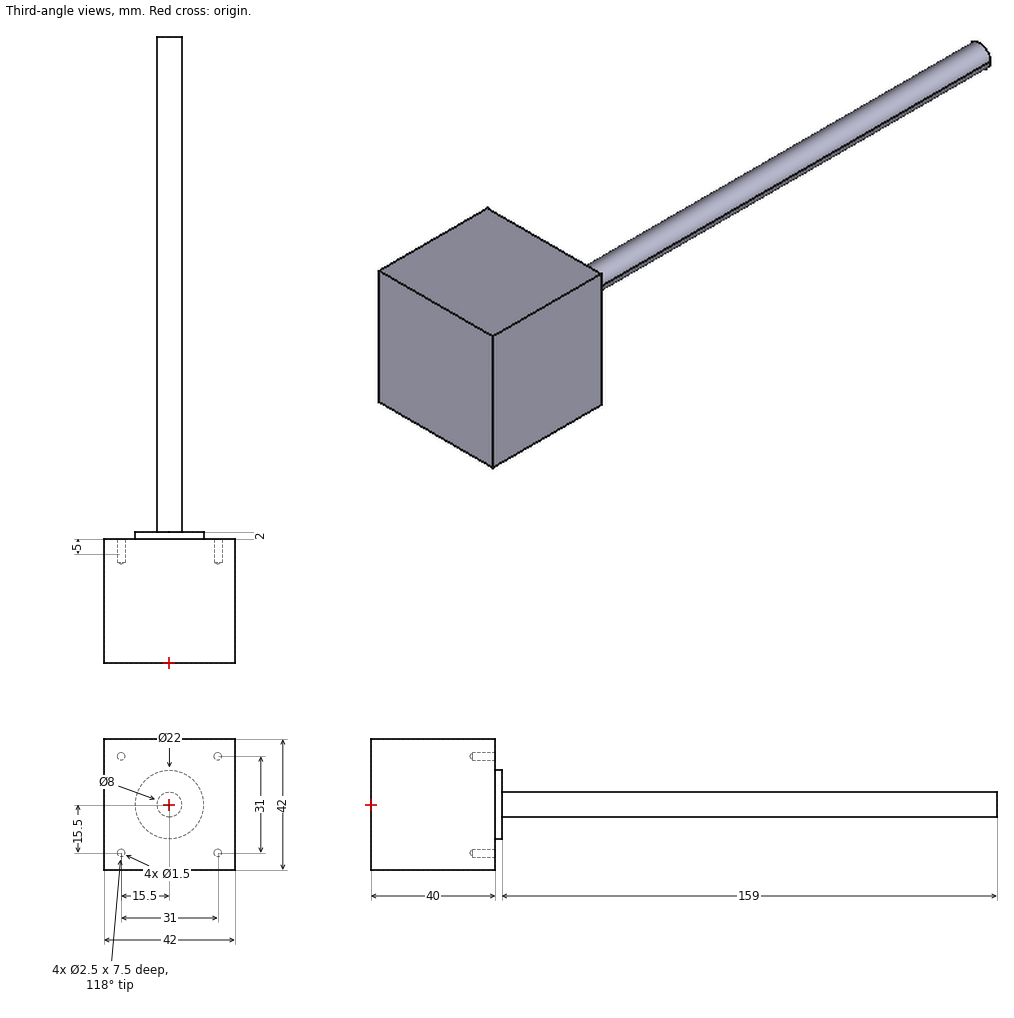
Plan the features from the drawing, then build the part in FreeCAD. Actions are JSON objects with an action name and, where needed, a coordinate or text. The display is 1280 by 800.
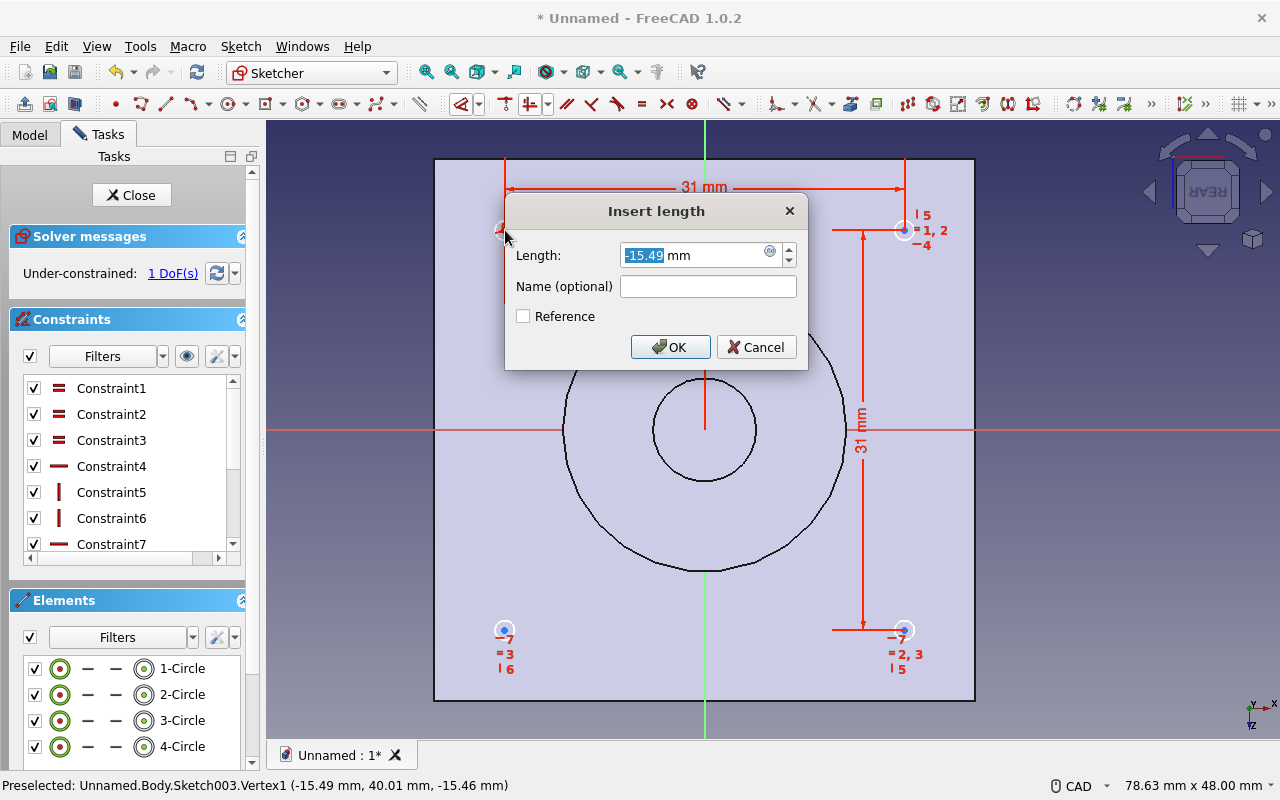
{"action": "type", "text": "-15.5"}
{"action": "key", "text": "Return"}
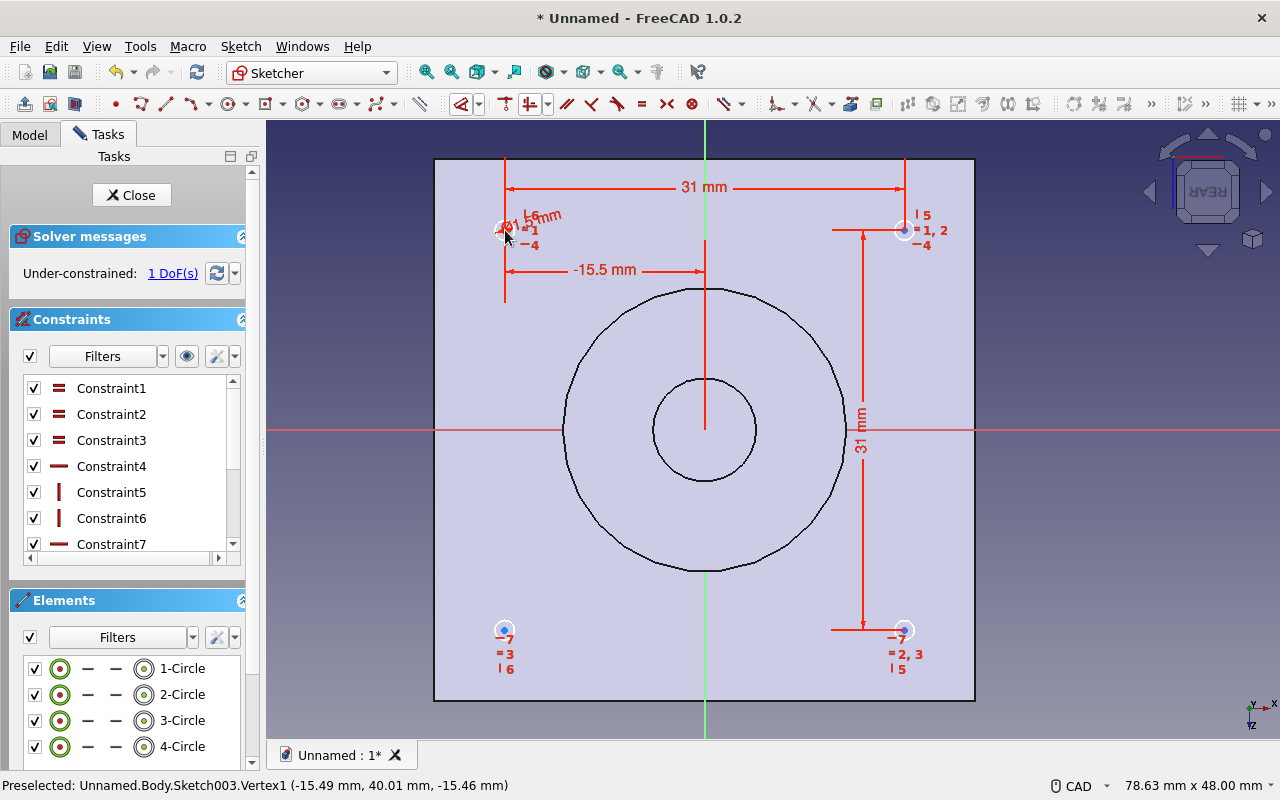
{"action": "left_click", "coordinate": [505, 230]}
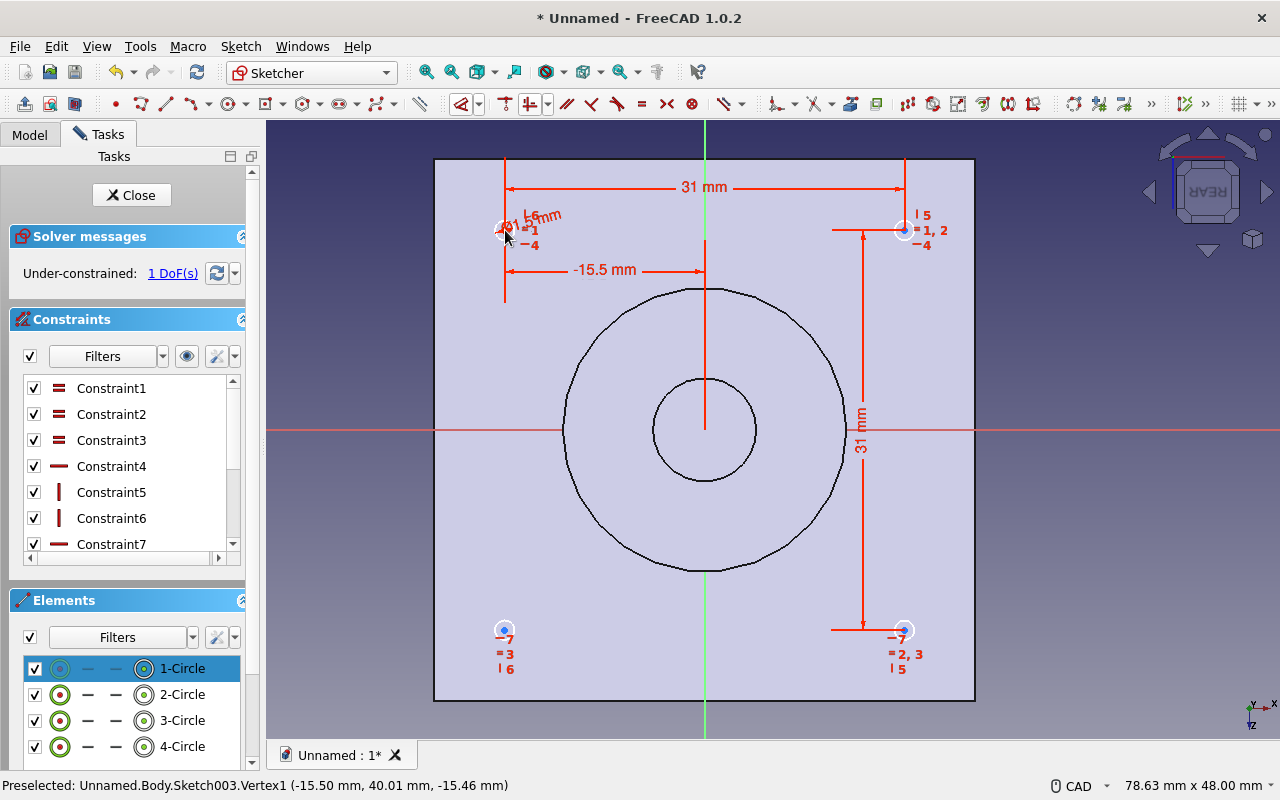
{"action": "key", "text": "i"}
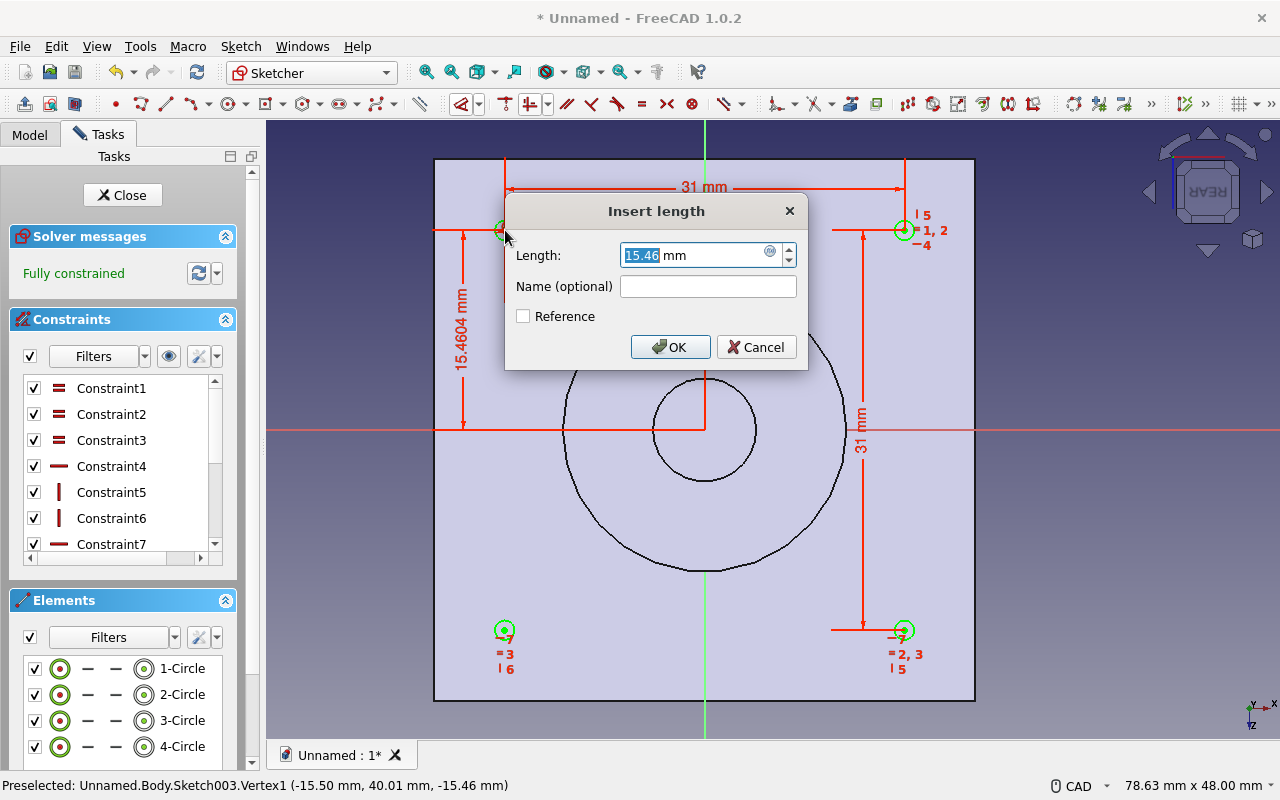
{"action": "type", "text": "15.5"}
{"action": "key", "text": "Return"}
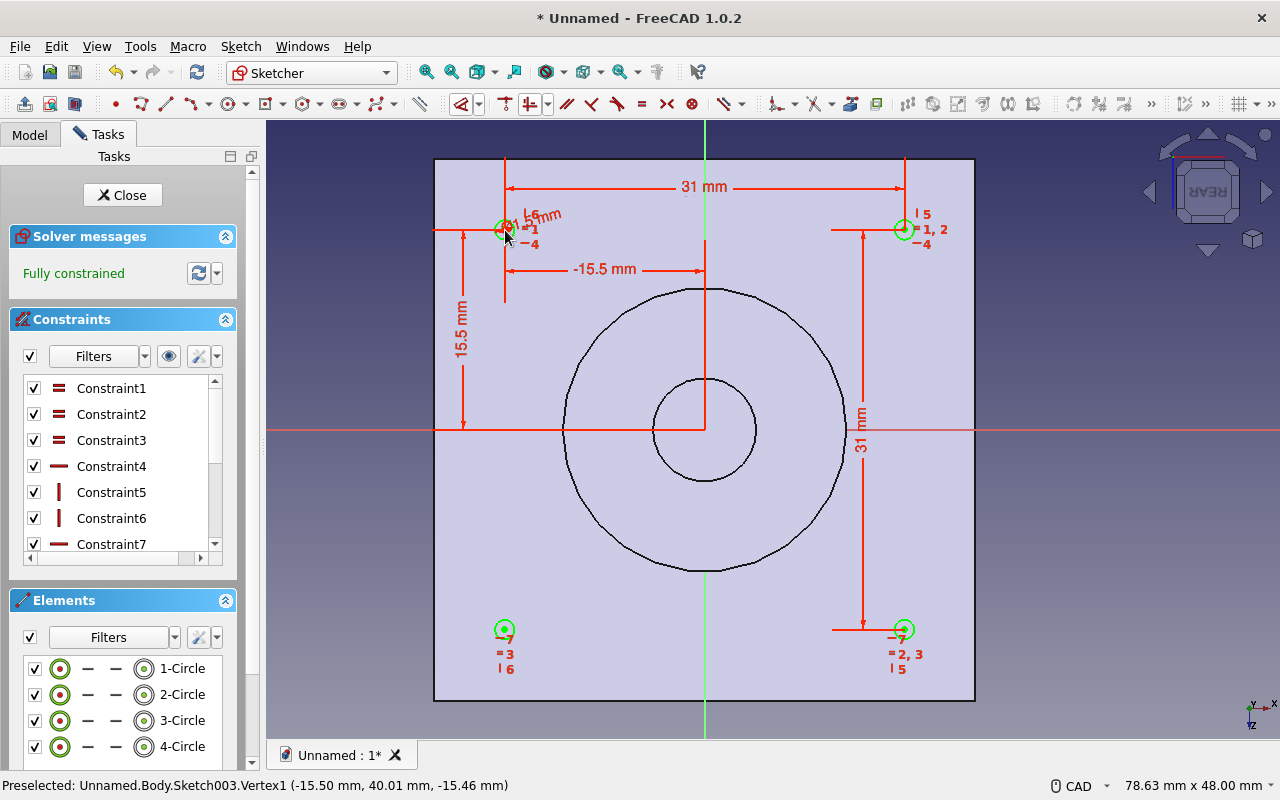
{"action": "left_click", "coordinate": [123, 195]}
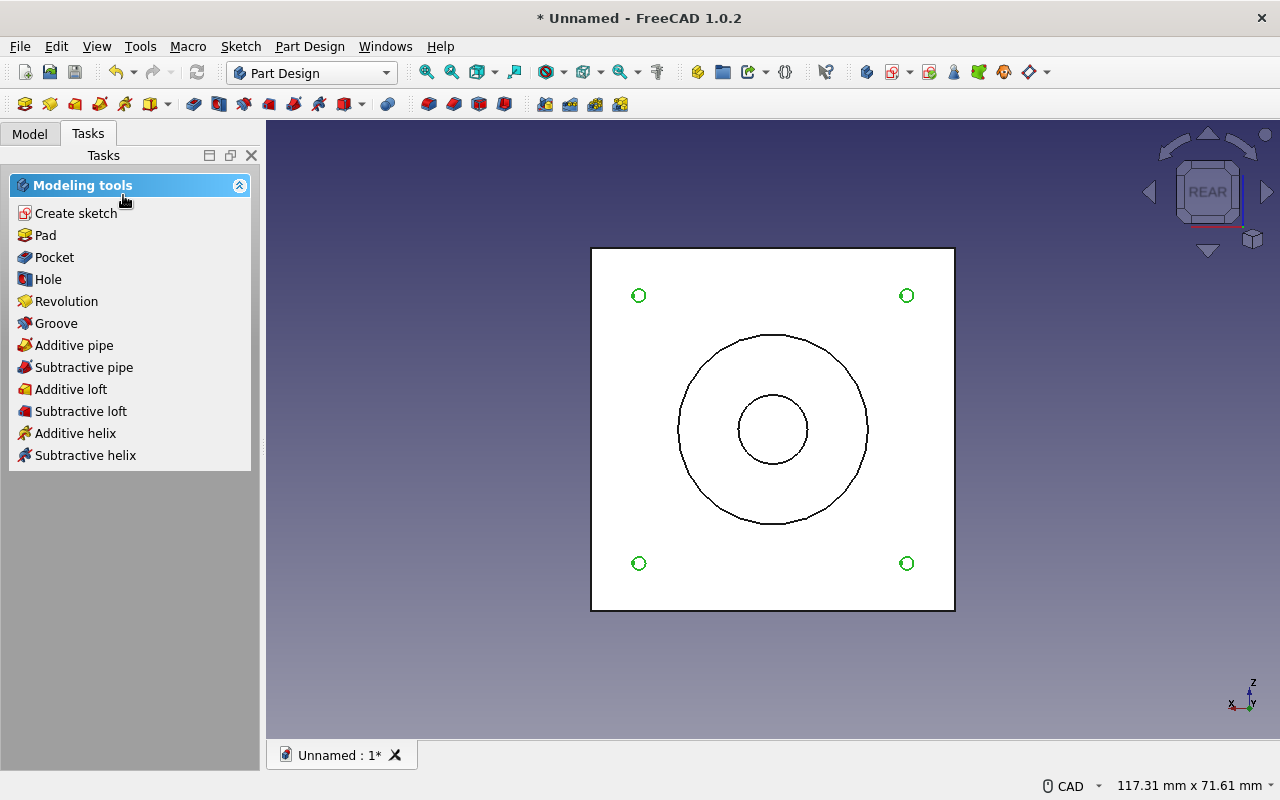
{"action": "left_click", "coordinate": [194, 104]}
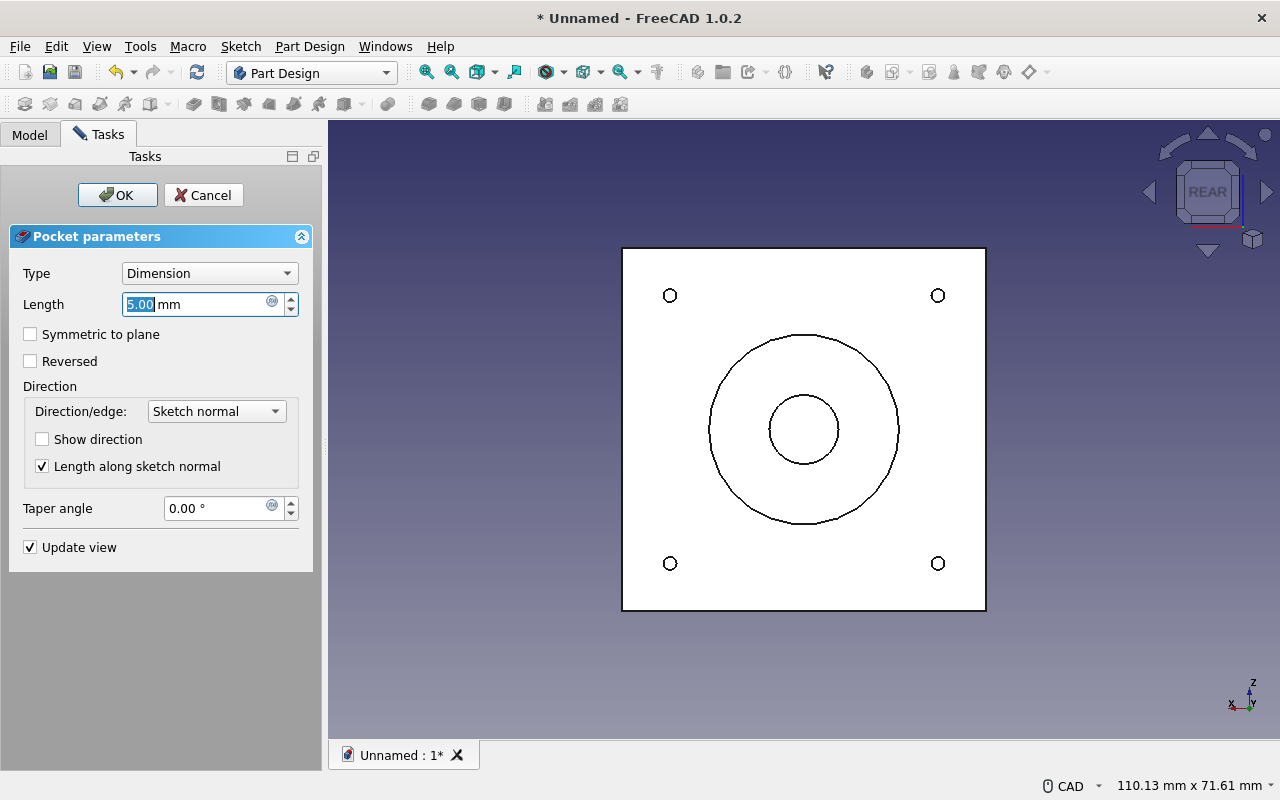
{"action": "type", "text": "5"}
{"action": "key", "text": "Tab"}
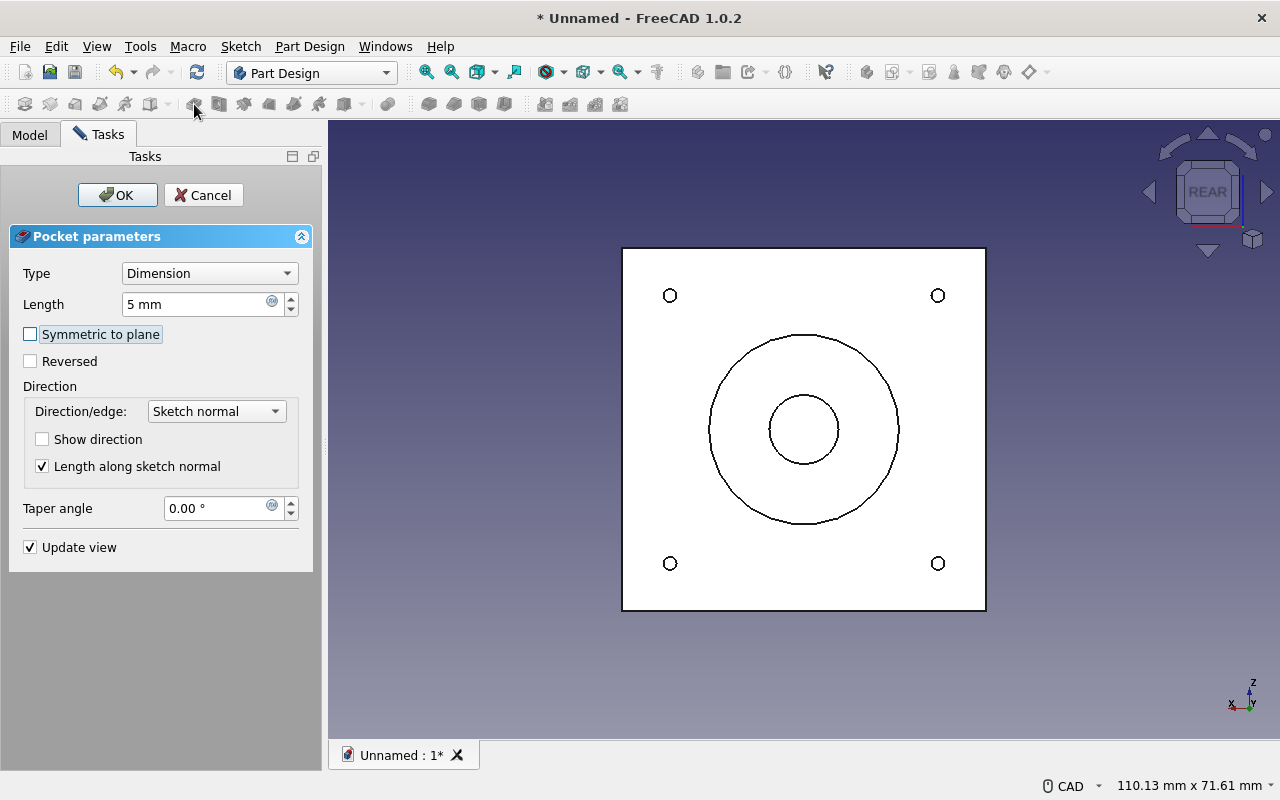
{"action": "left_click", "coordinate": [118, 195]}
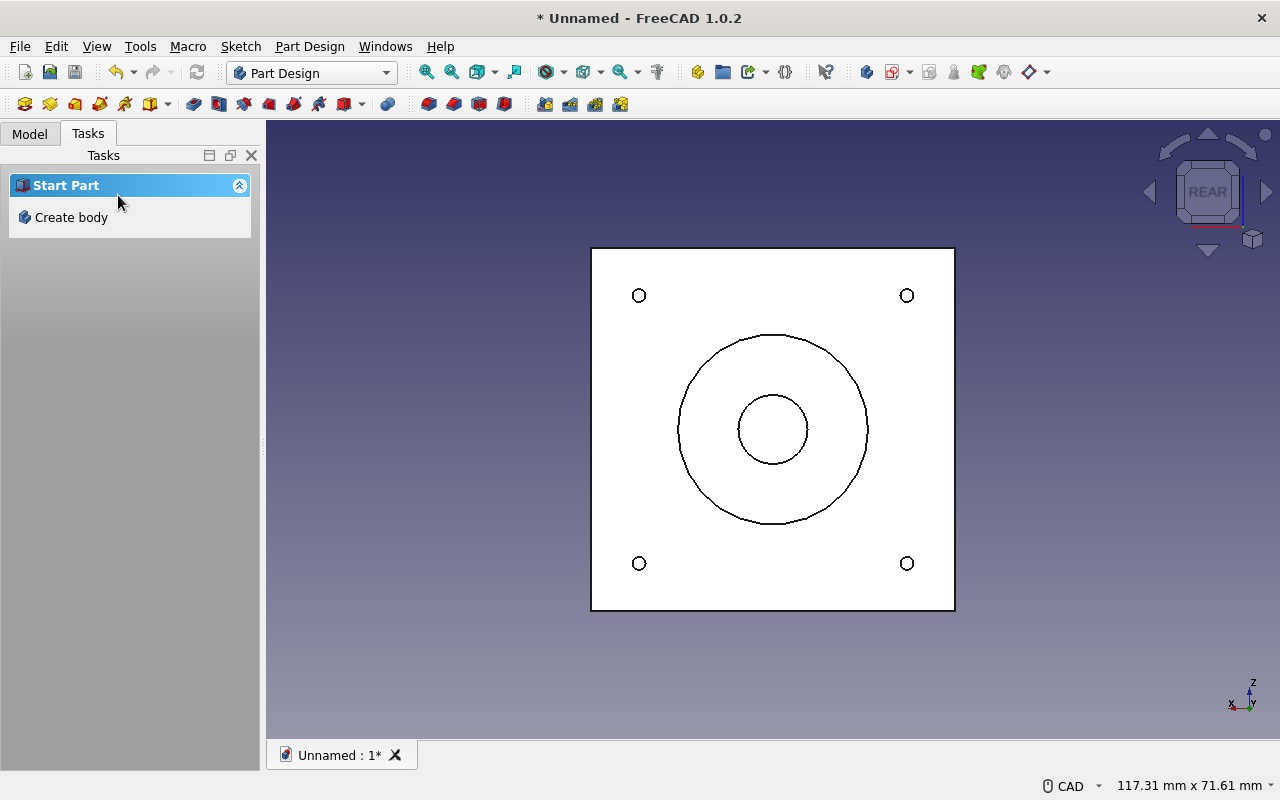
{"action": "left_click", "coordinate": [669, 325]}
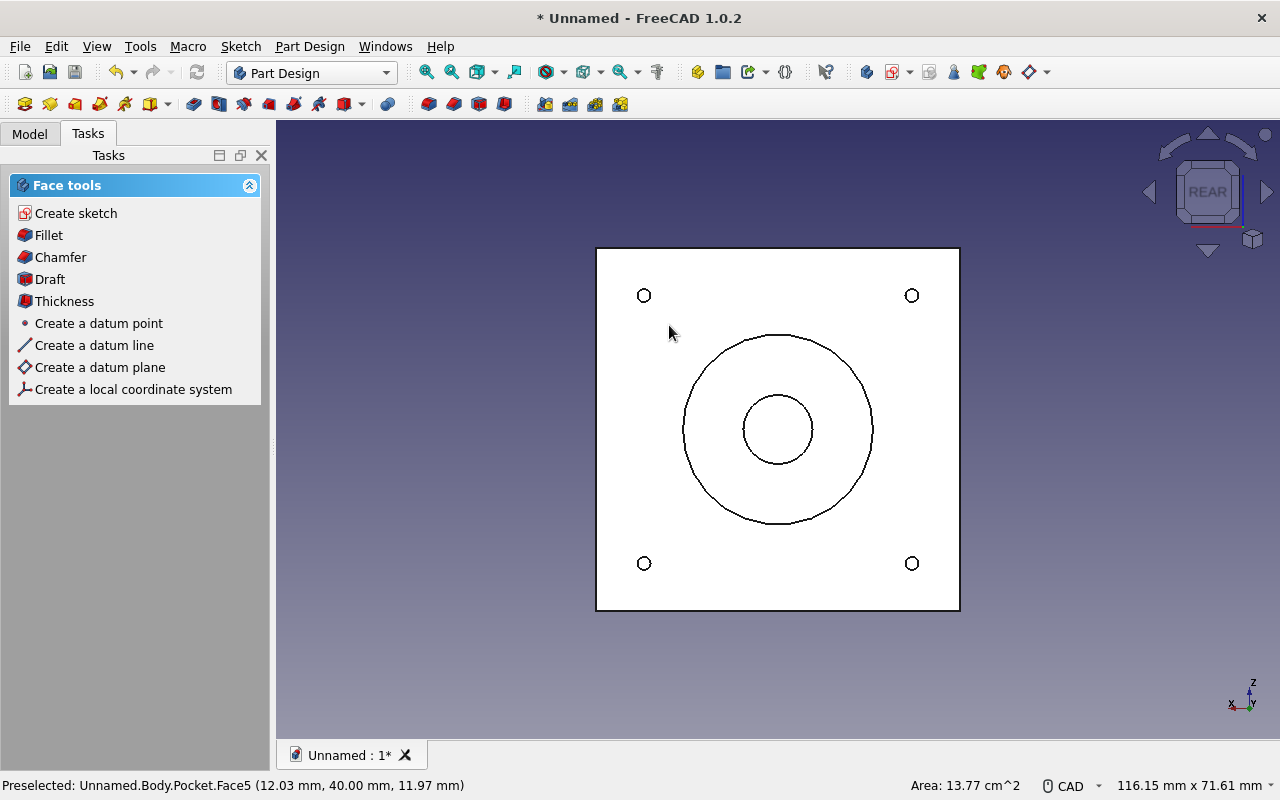
{"action": "left_click", "coordinate": [892, 72]}